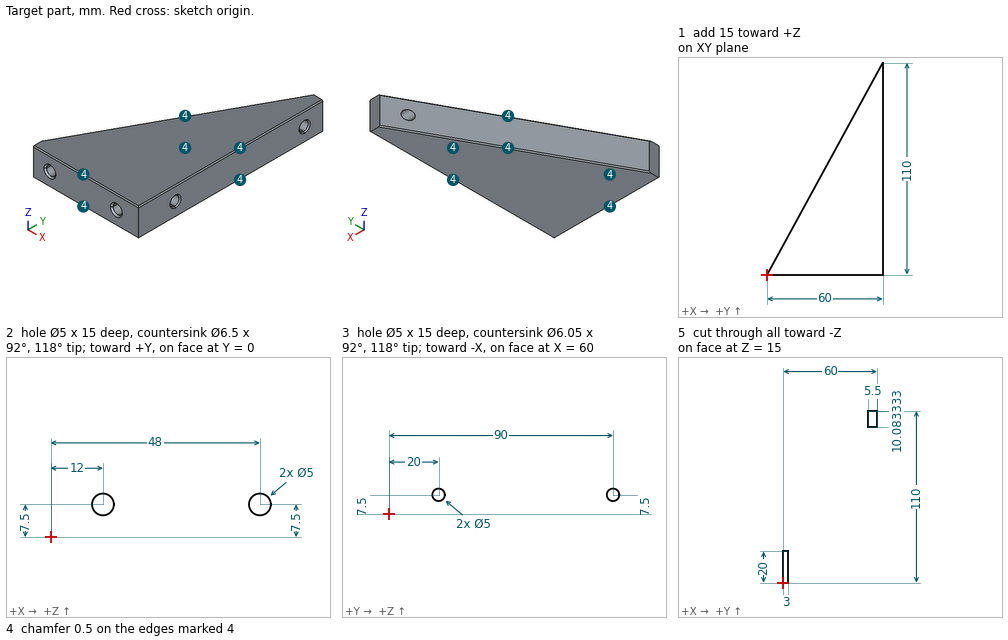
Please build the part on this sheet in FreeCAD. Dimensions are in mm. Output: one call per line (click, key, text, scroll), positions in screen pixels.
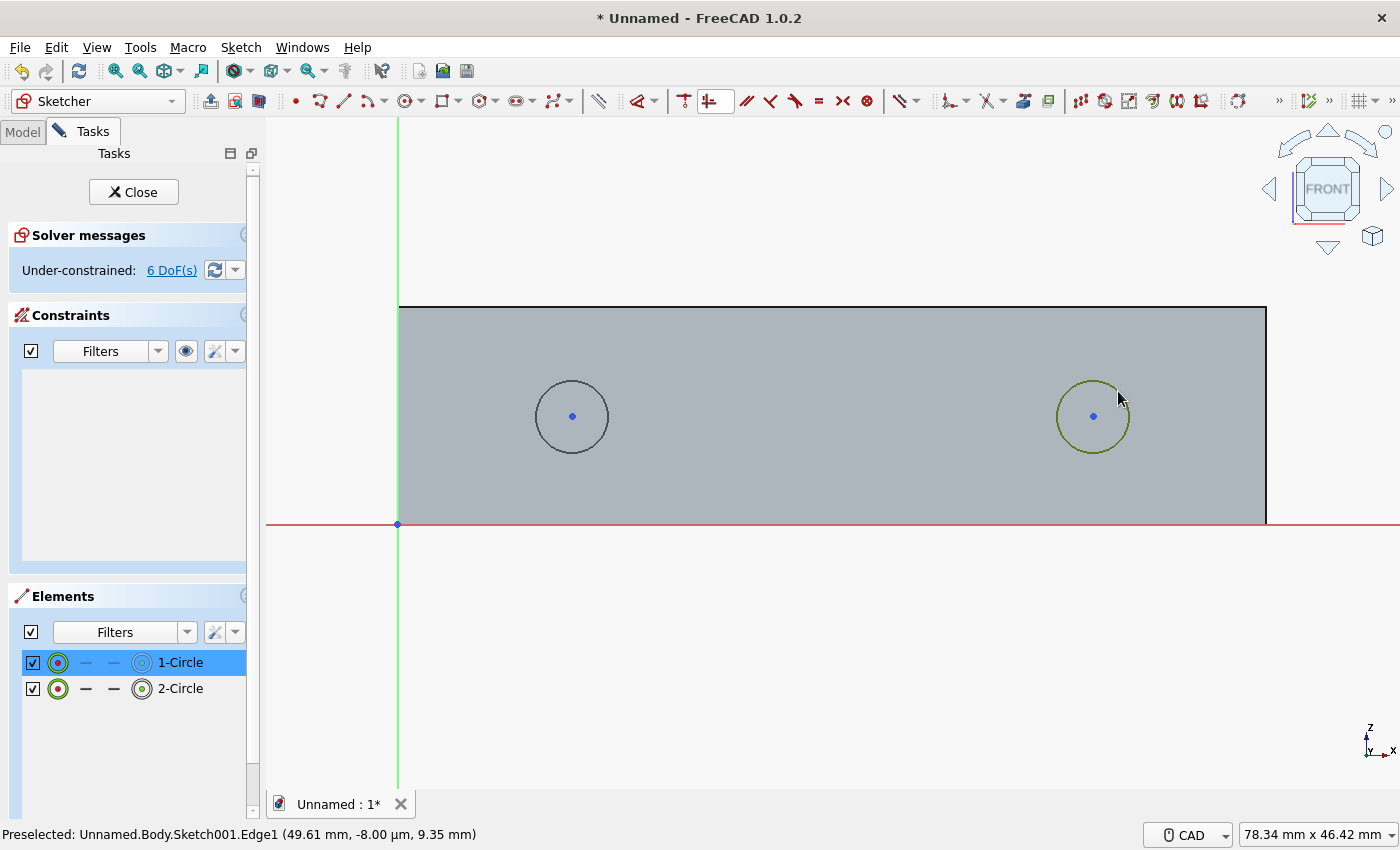
click(597, 391)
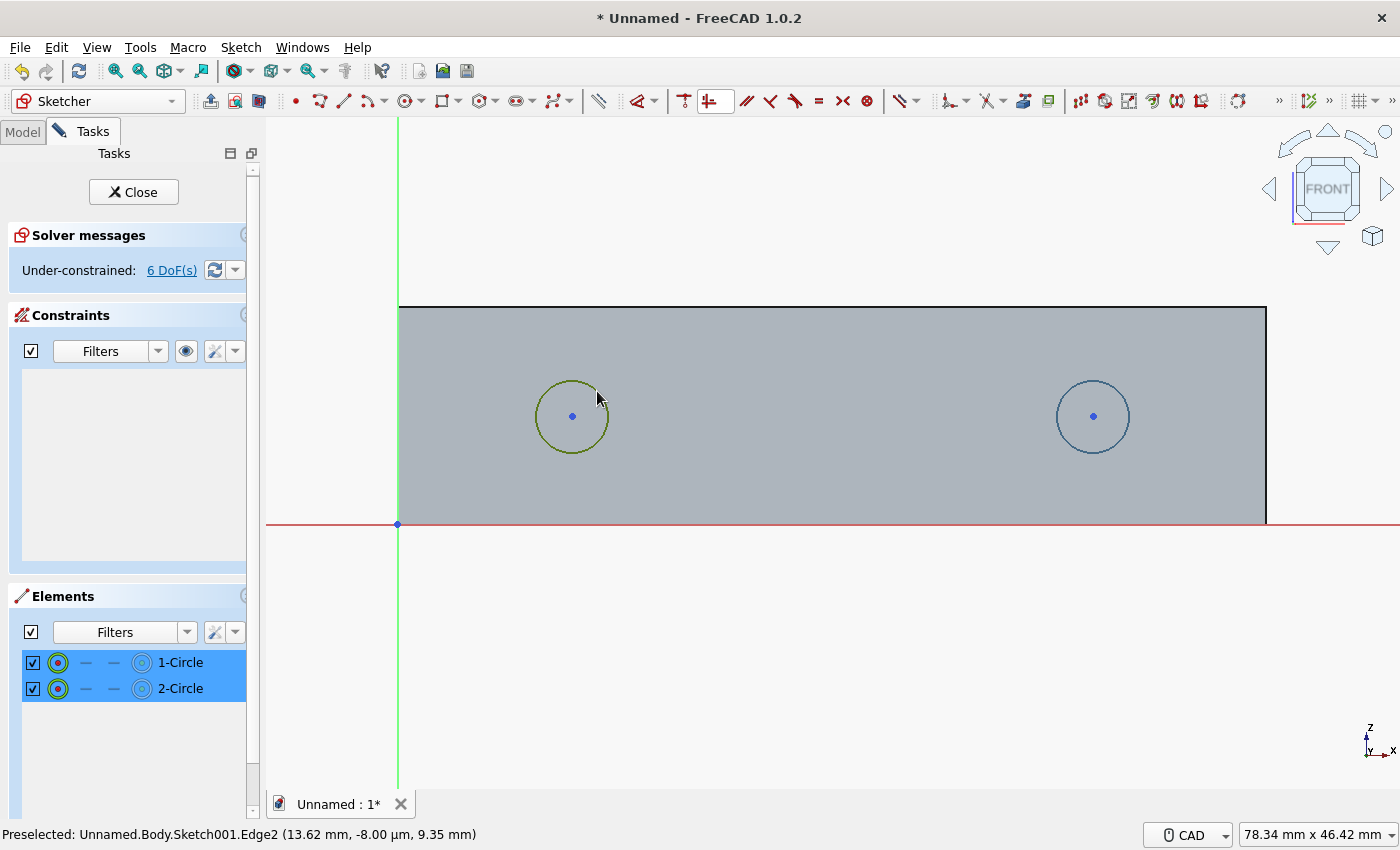
click(820, 102)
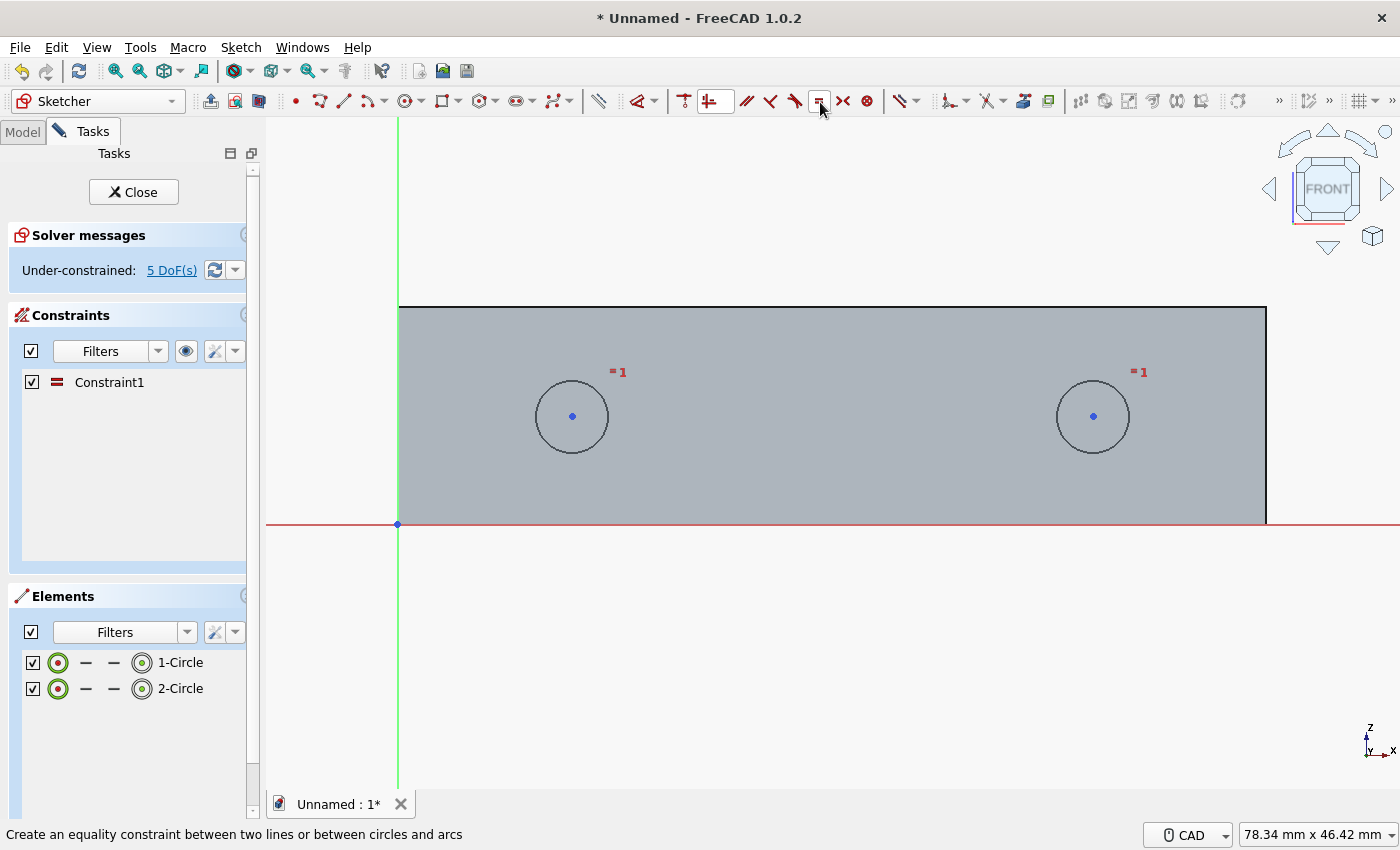
click(638, 102)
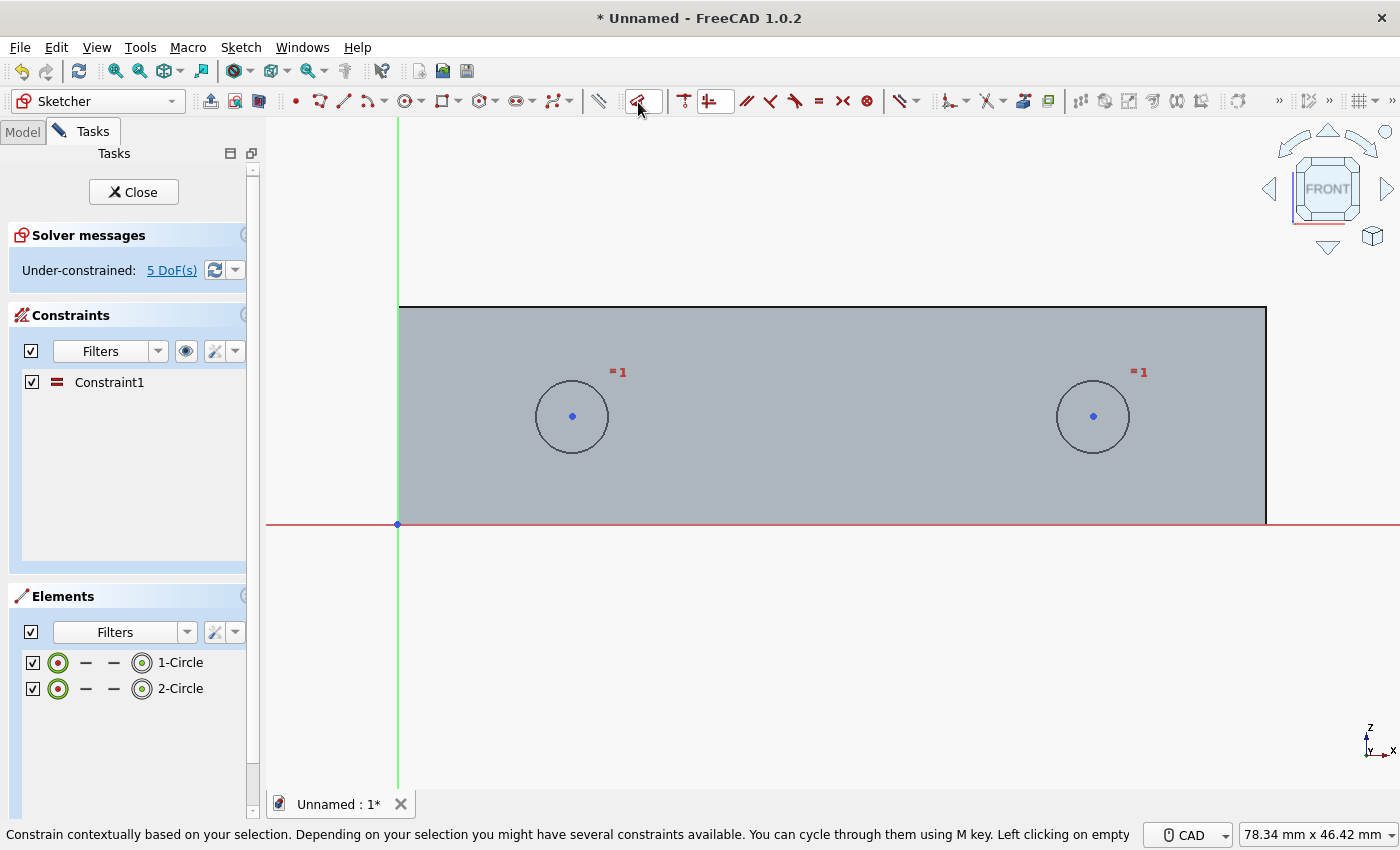
click(1118, 391)
click(1140, 368)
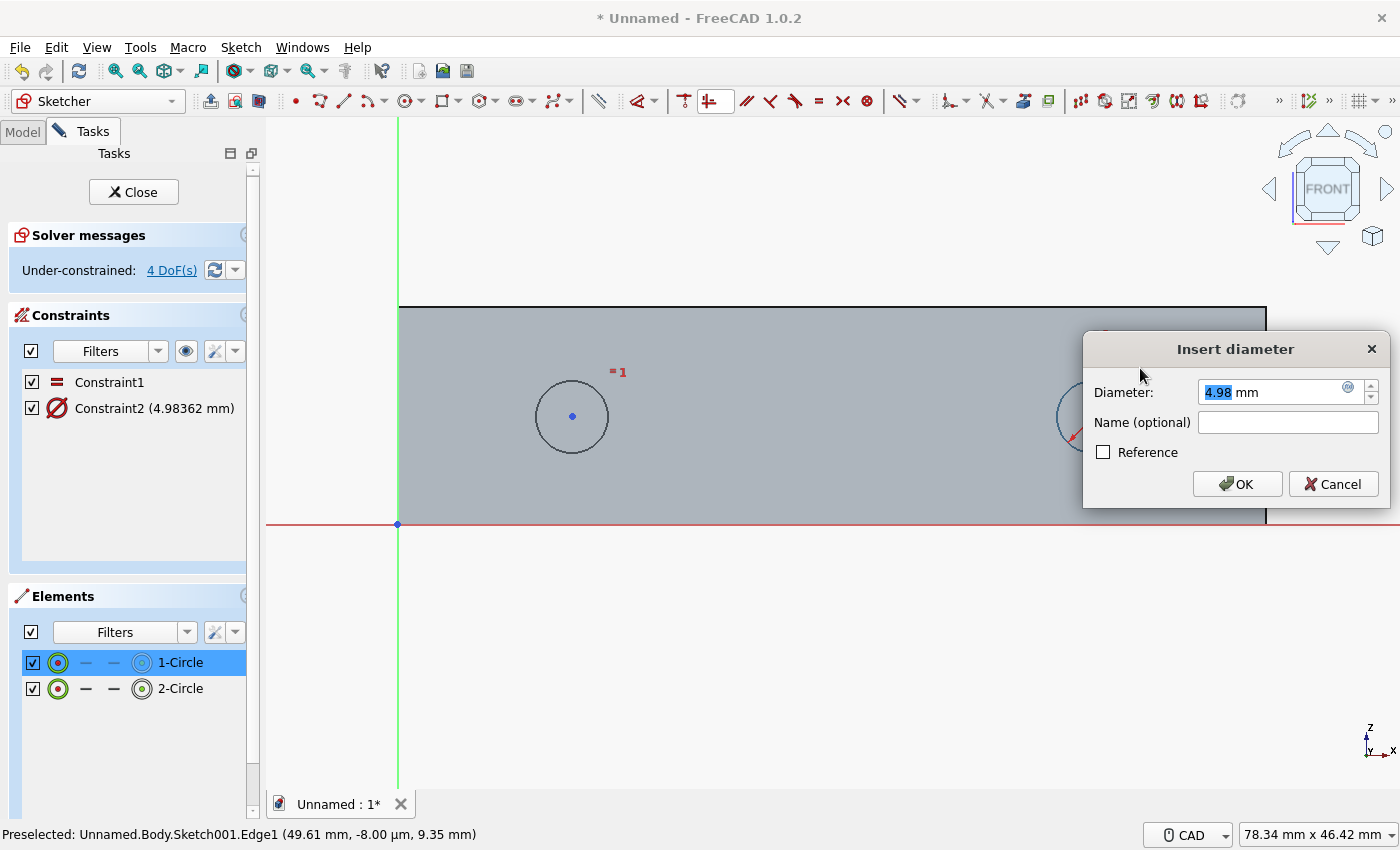
text(5)
key(Return)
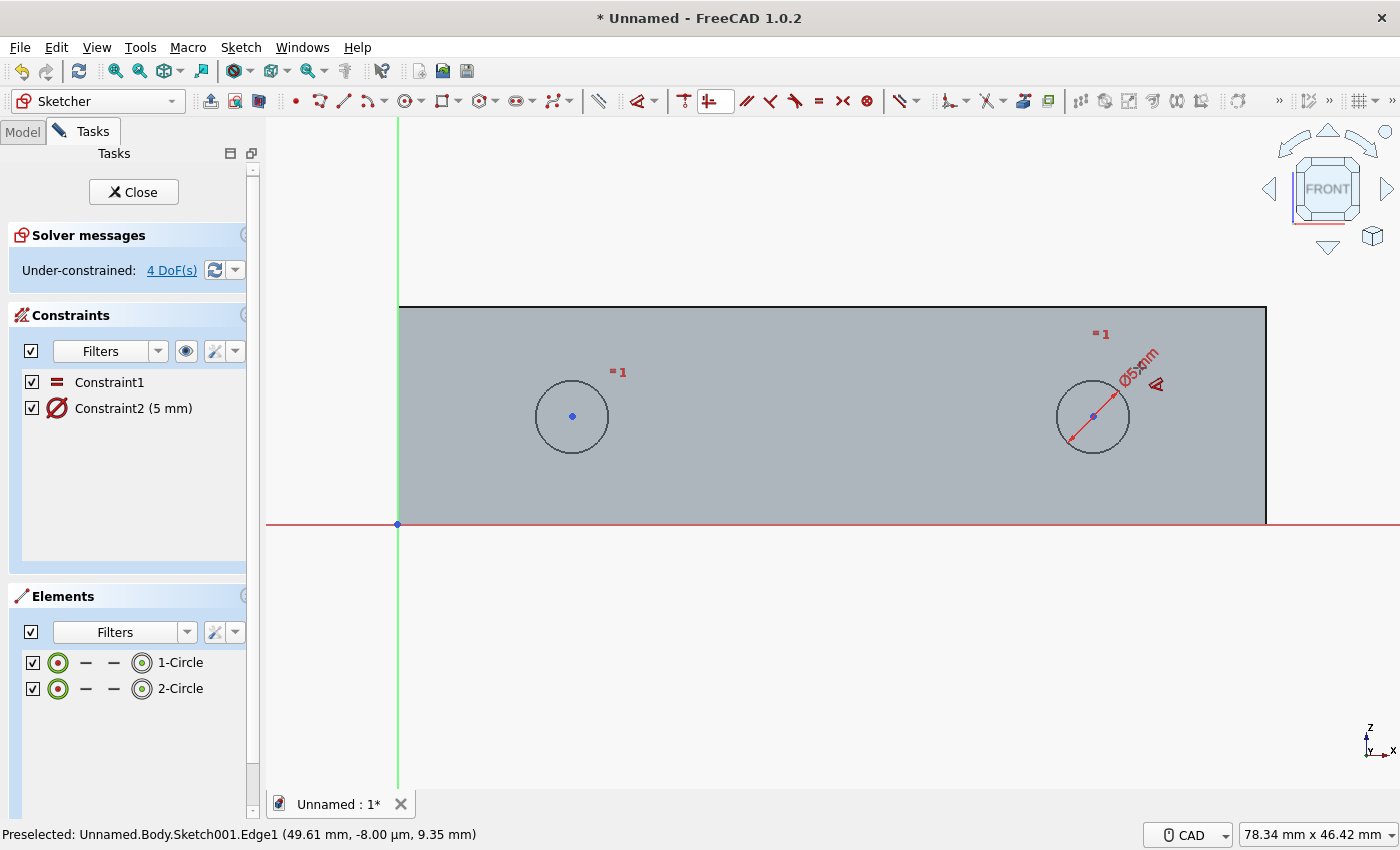
click(1093, 417)
click(745, 559)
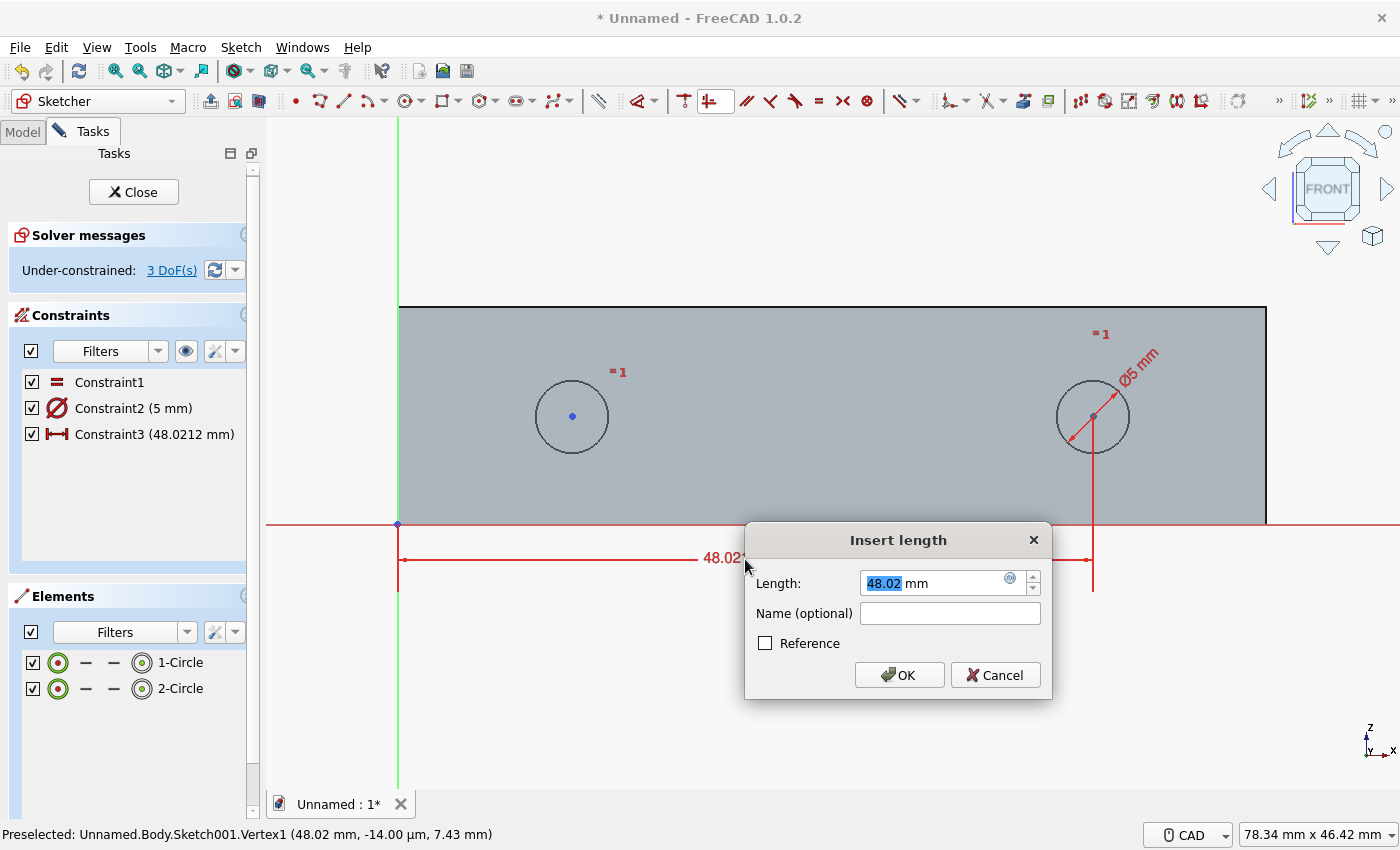
text(48)
key(Return)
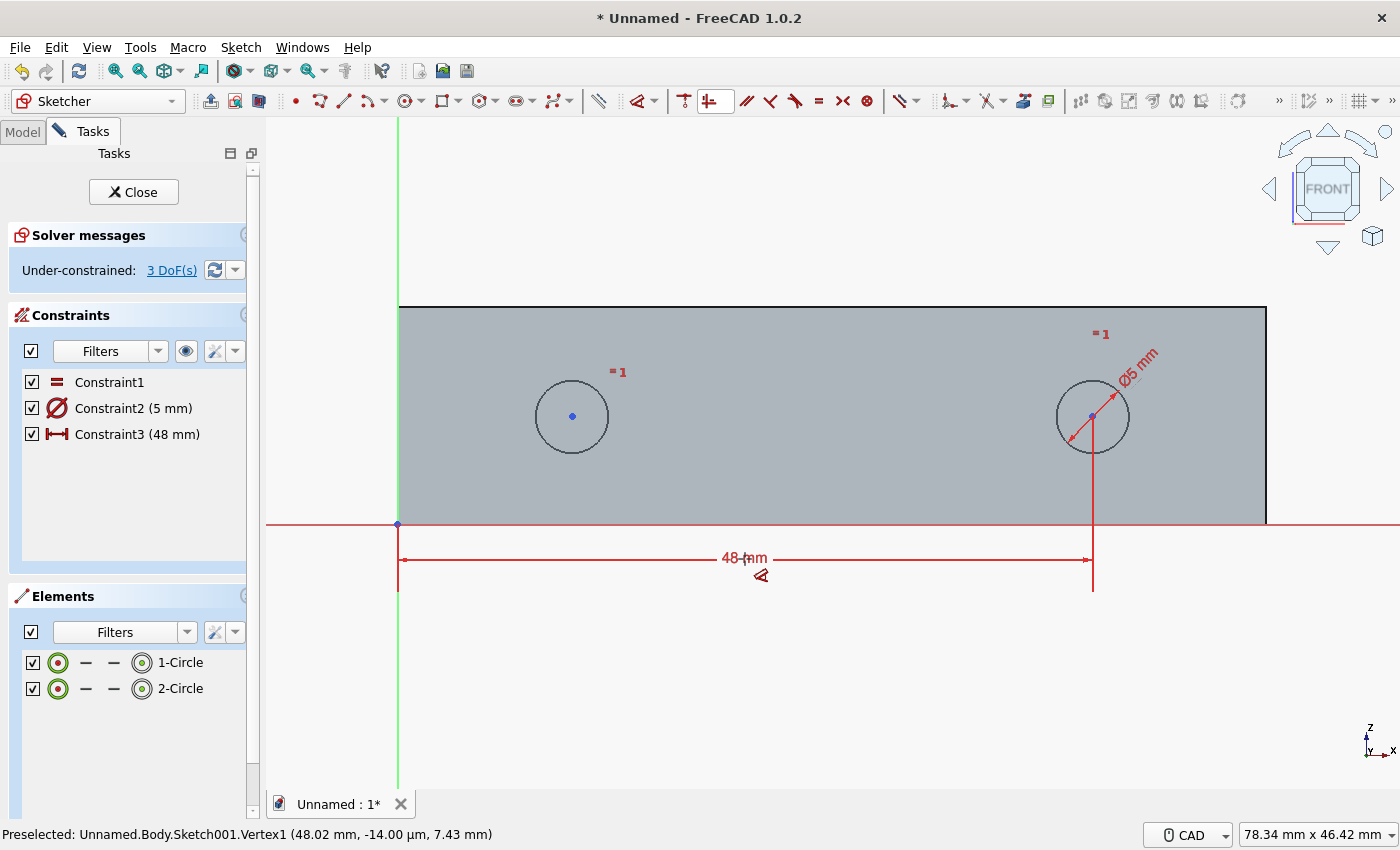
click(572, 417)
click(485, 559)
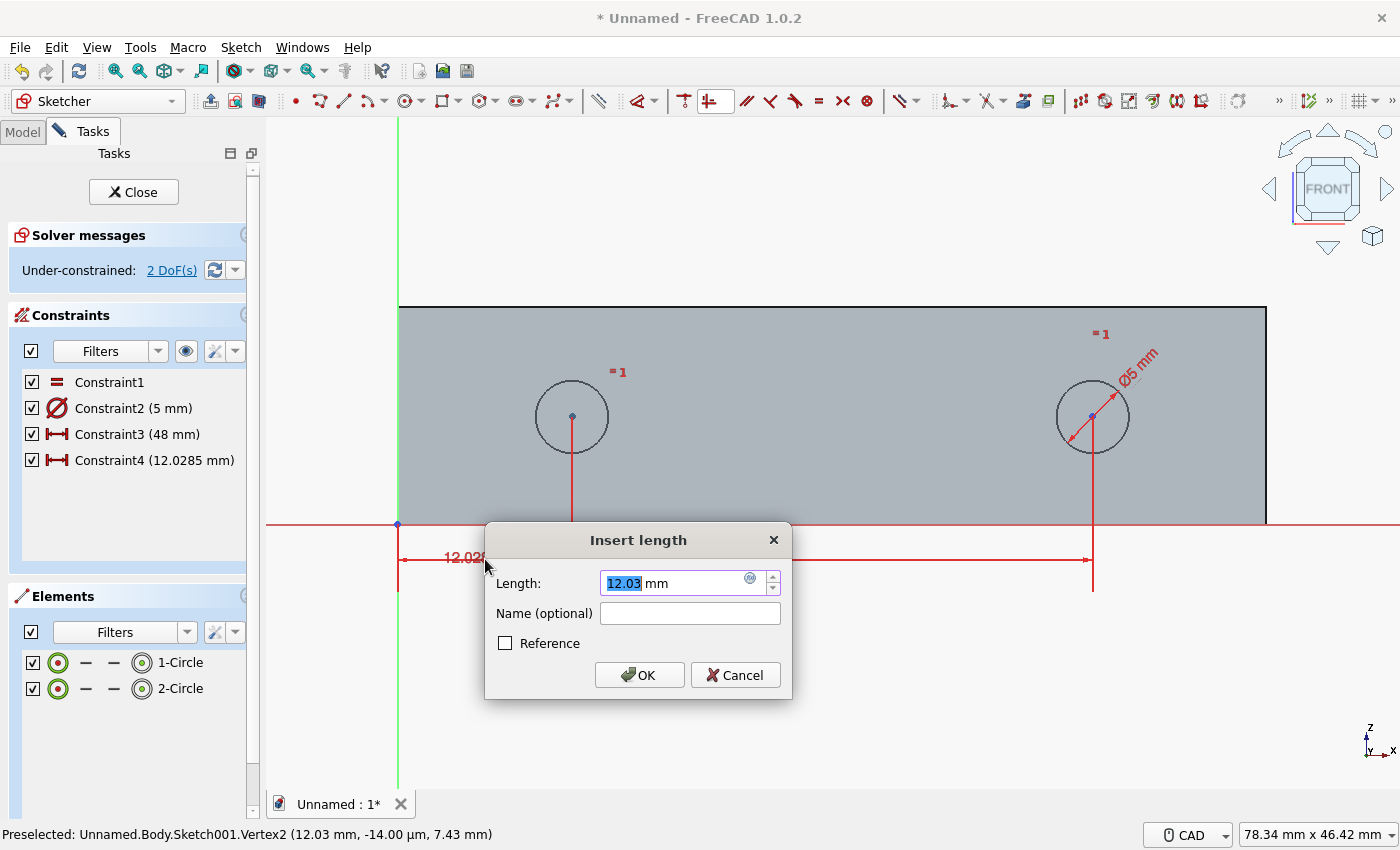
text(12)
key(Return)